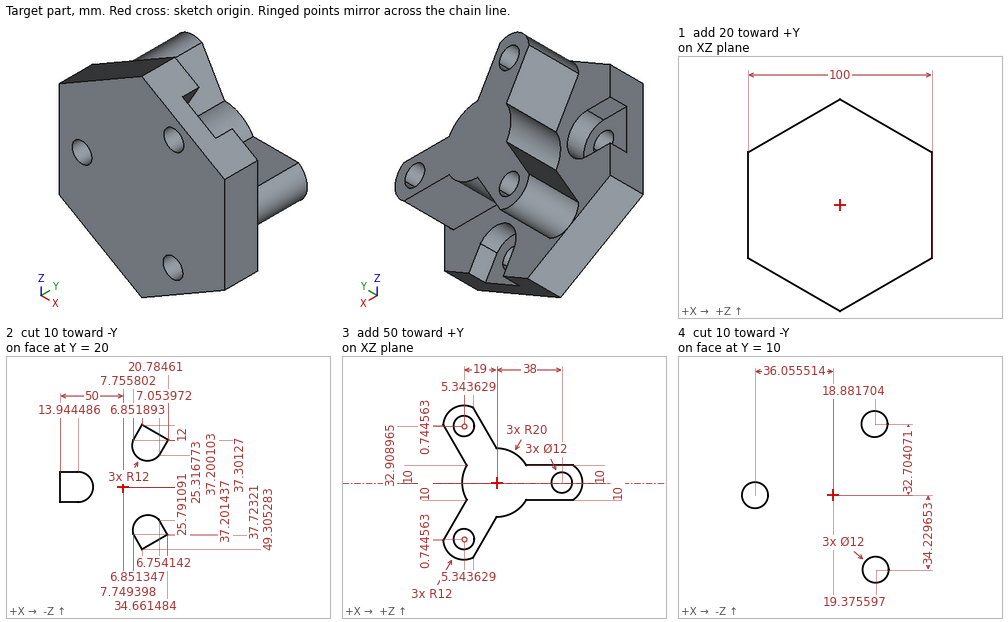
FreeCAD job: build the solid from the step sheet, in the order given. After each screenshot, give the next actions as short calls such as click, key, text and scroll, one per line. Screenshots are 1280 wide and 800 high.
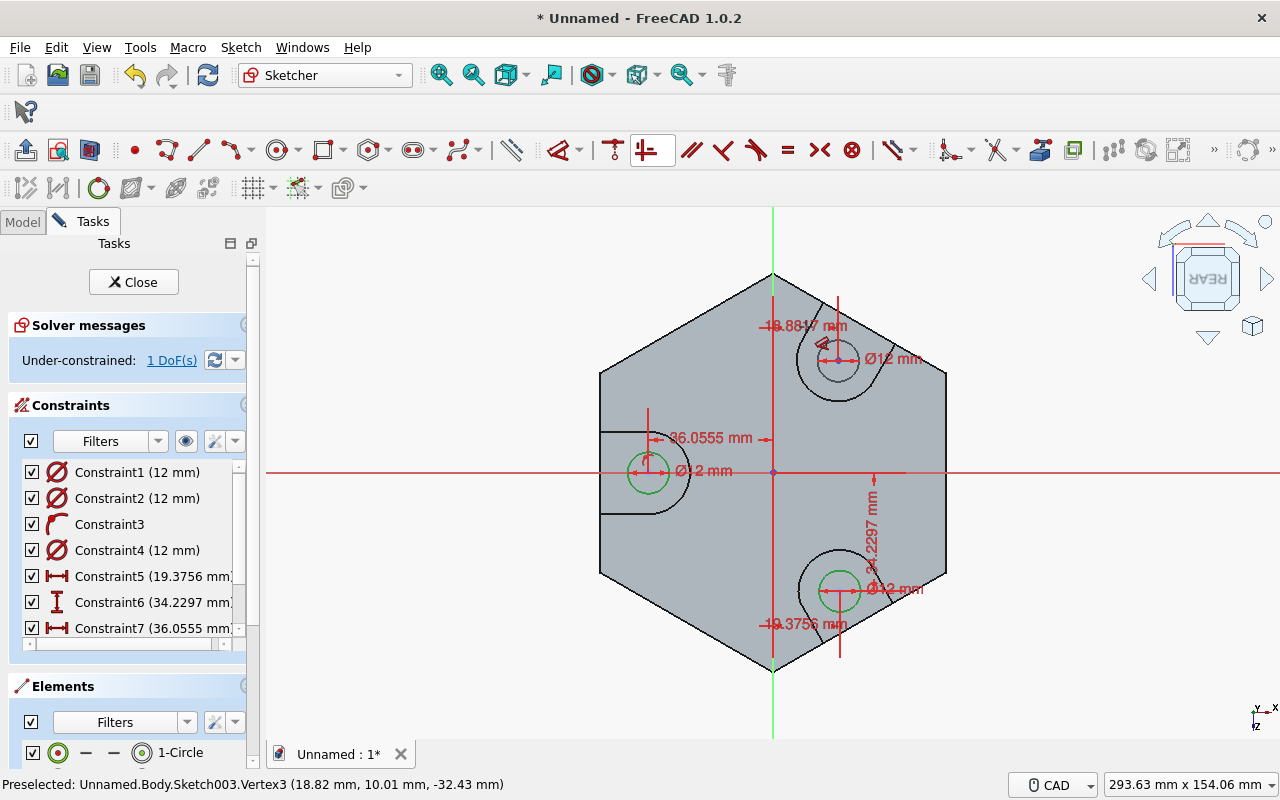
click(838, 361)
click(872, 417)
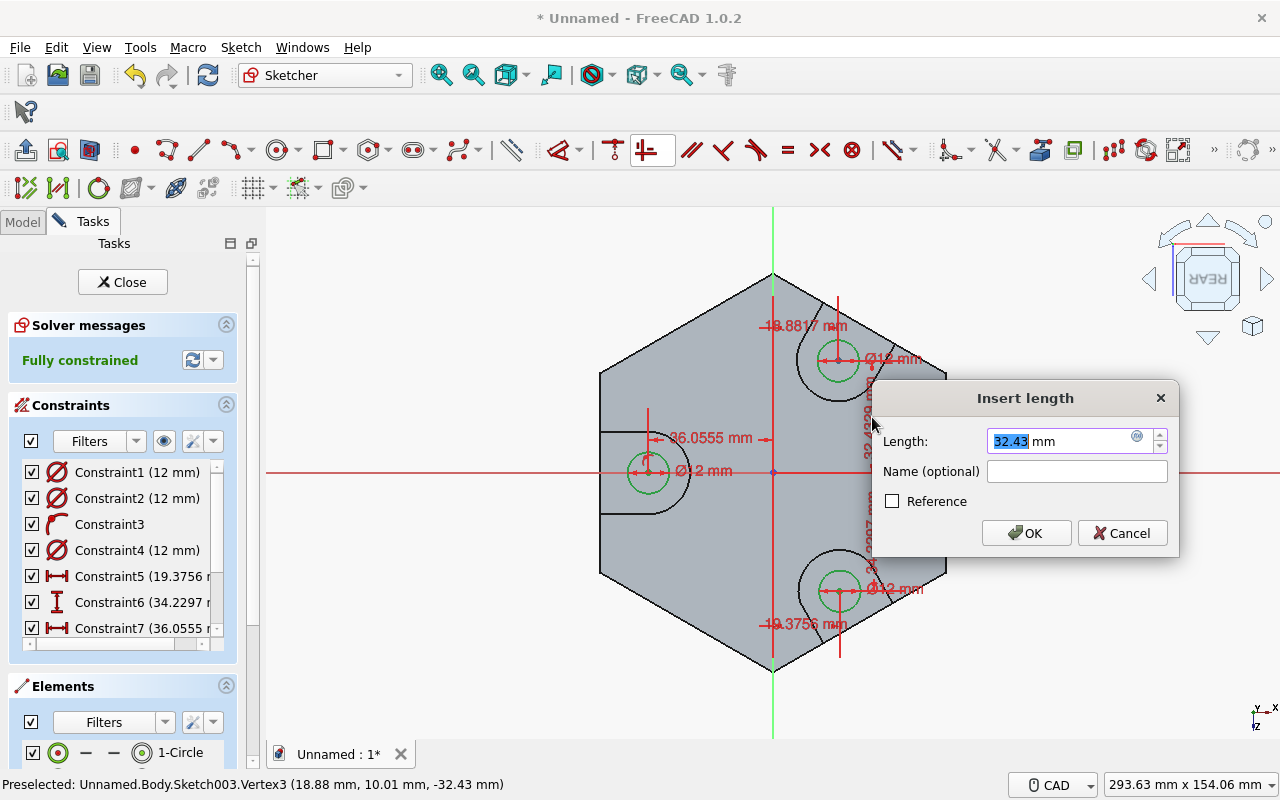
text(32.704071)
key(Return)
key(Escape)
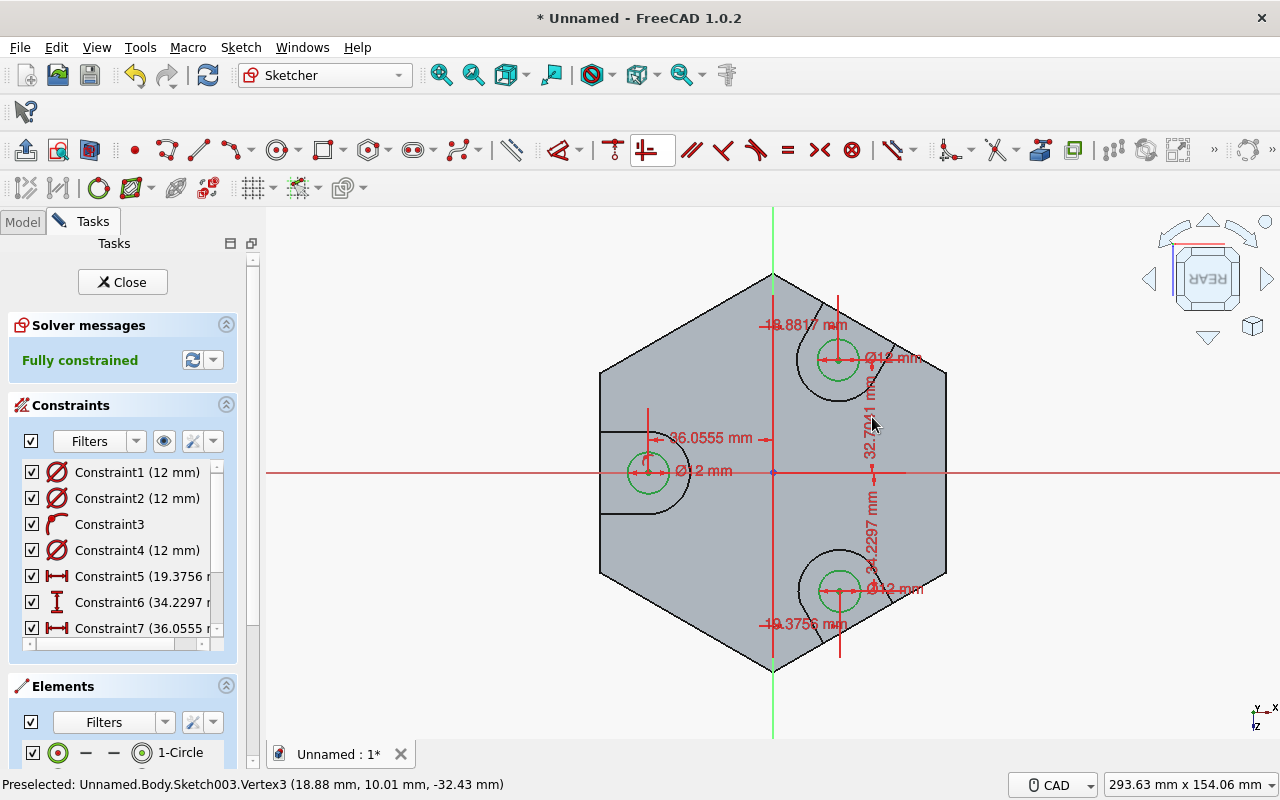
click(123, 282)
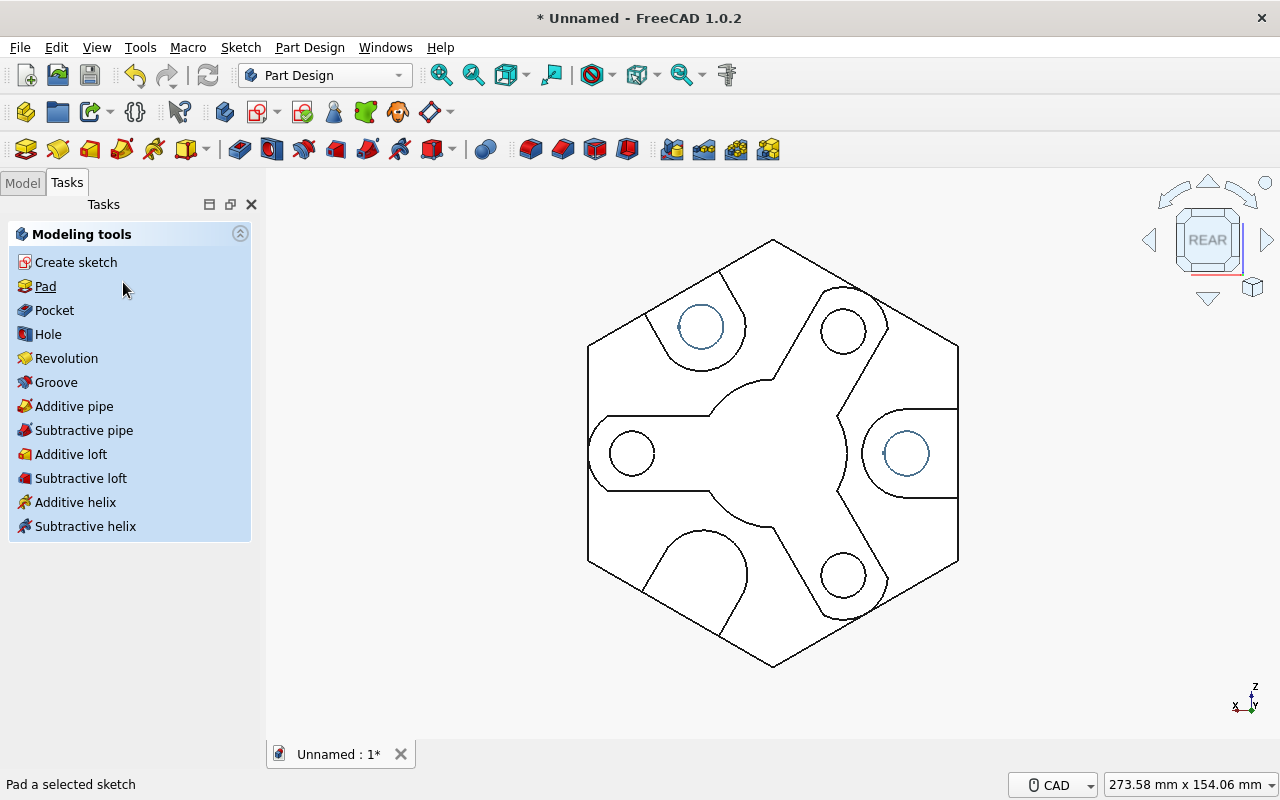
click(240, 150)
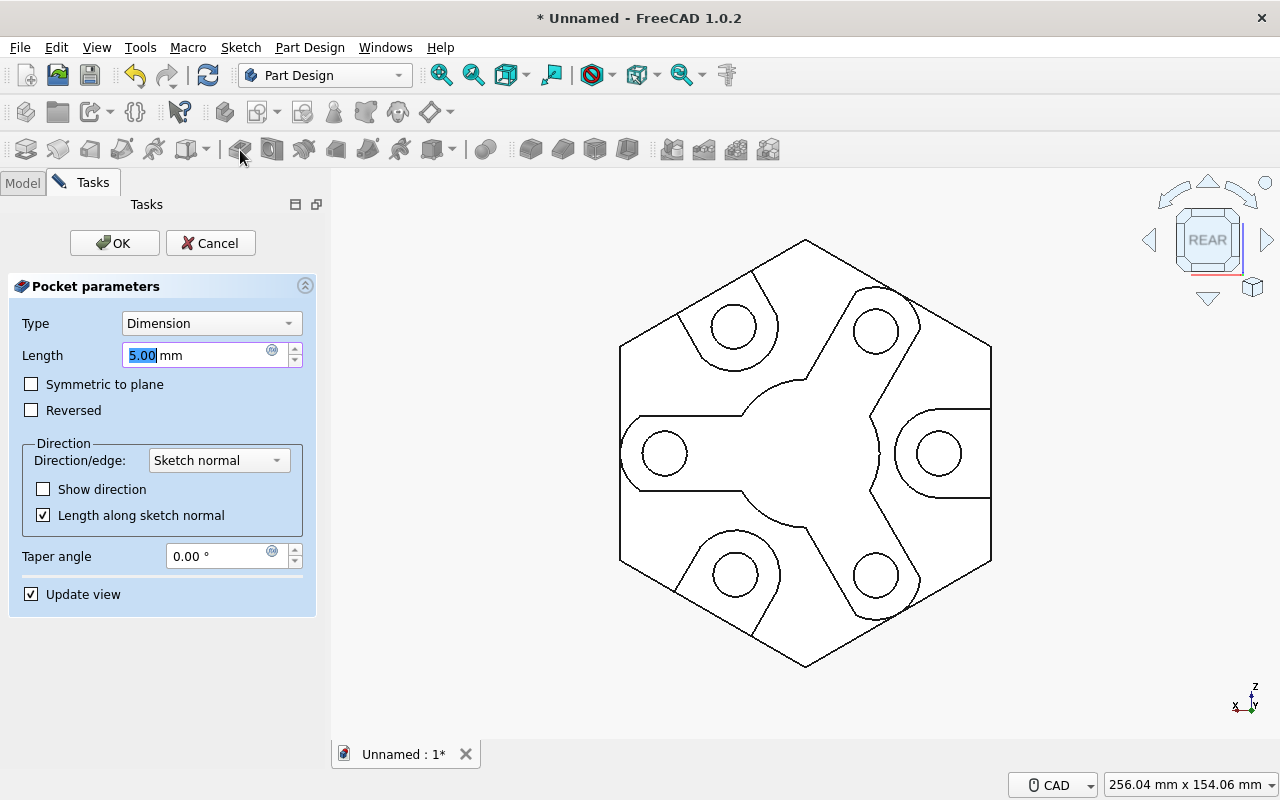
text(10)
key(Tab)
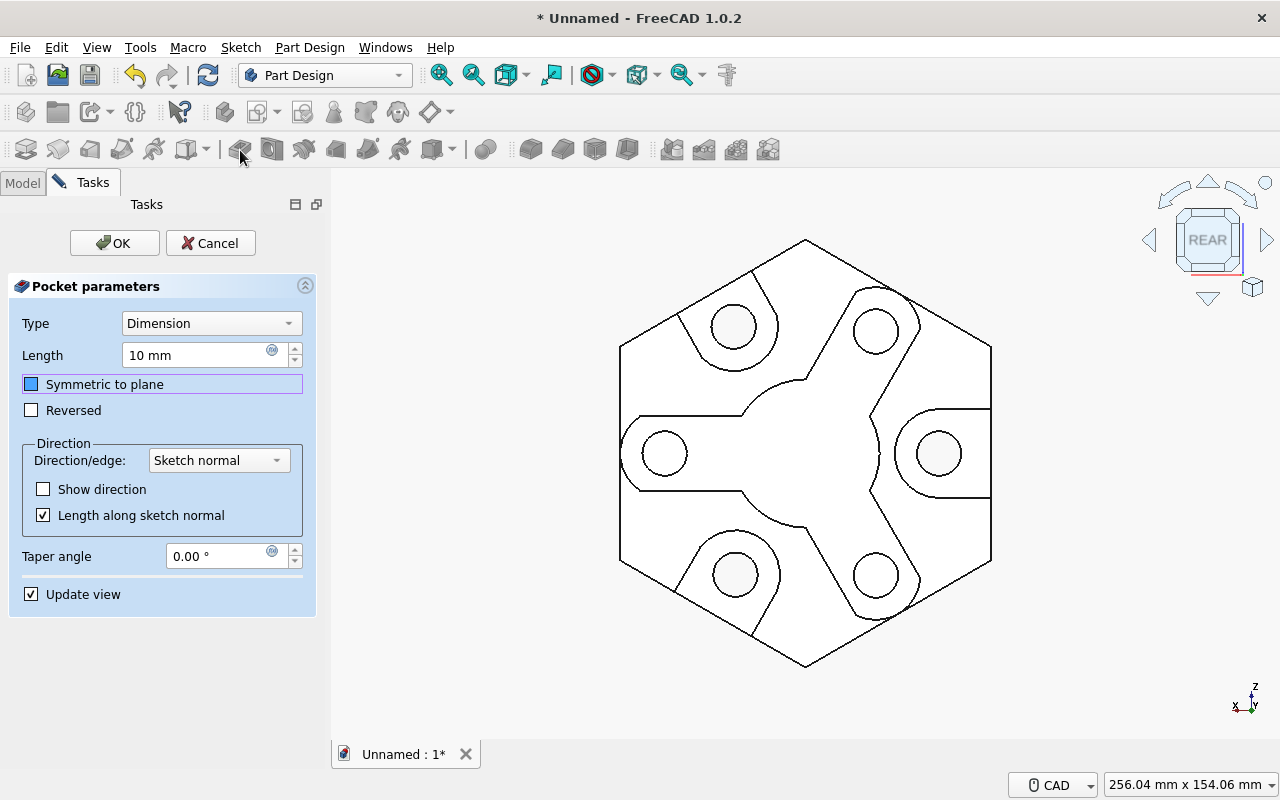
click(115, 243)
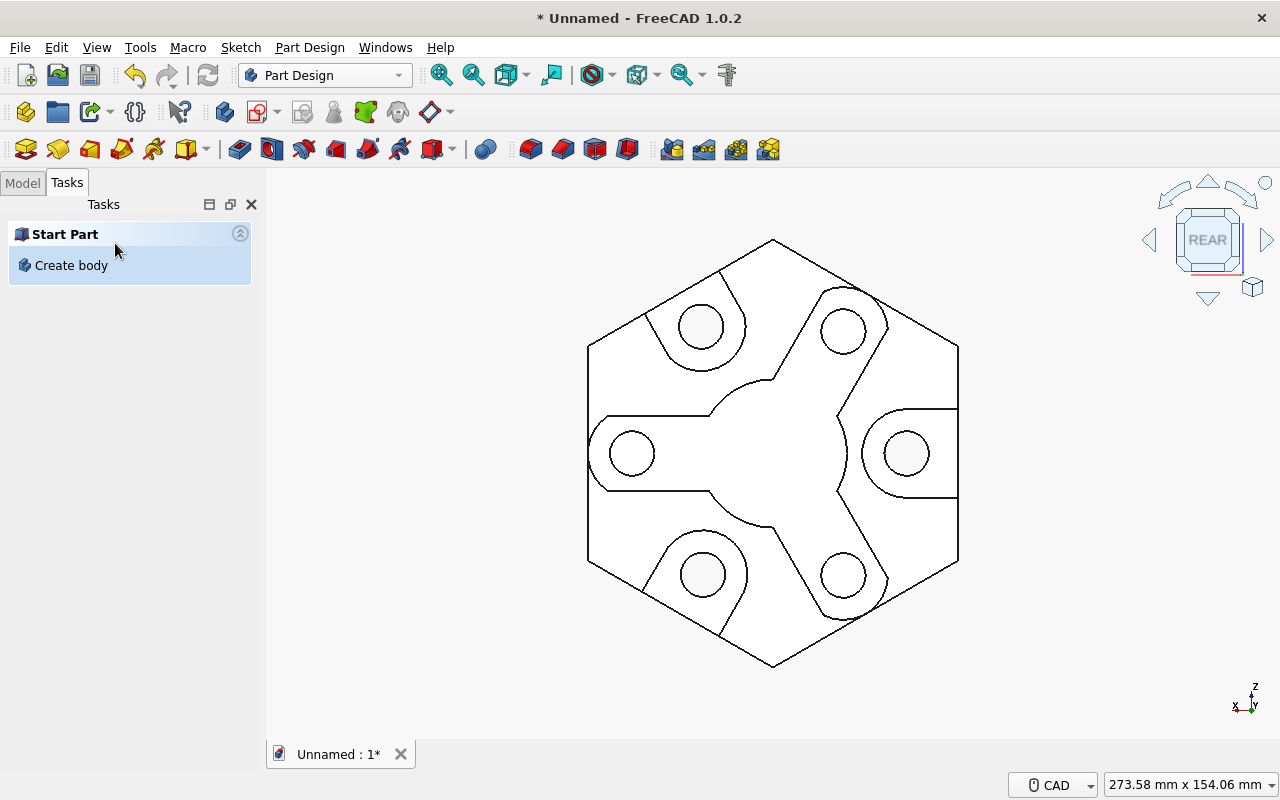
key(0)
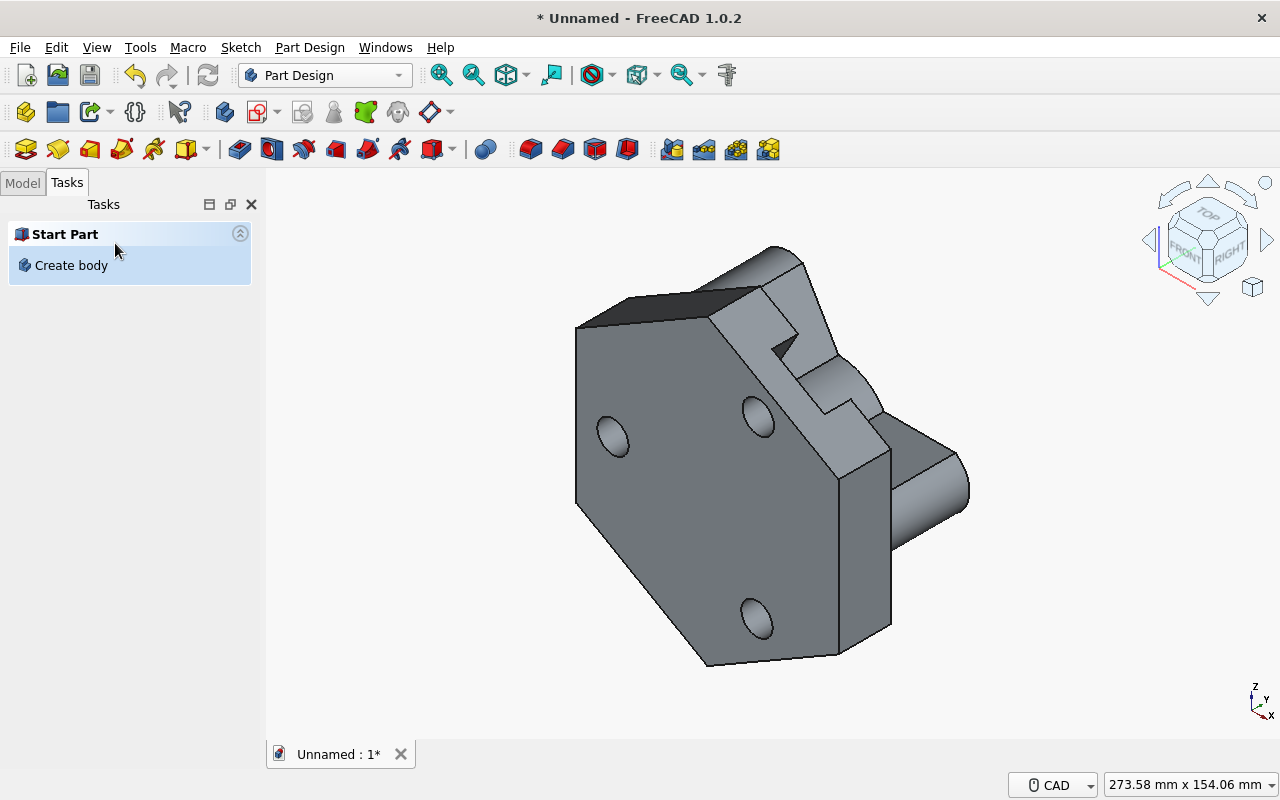
click(442, 76)